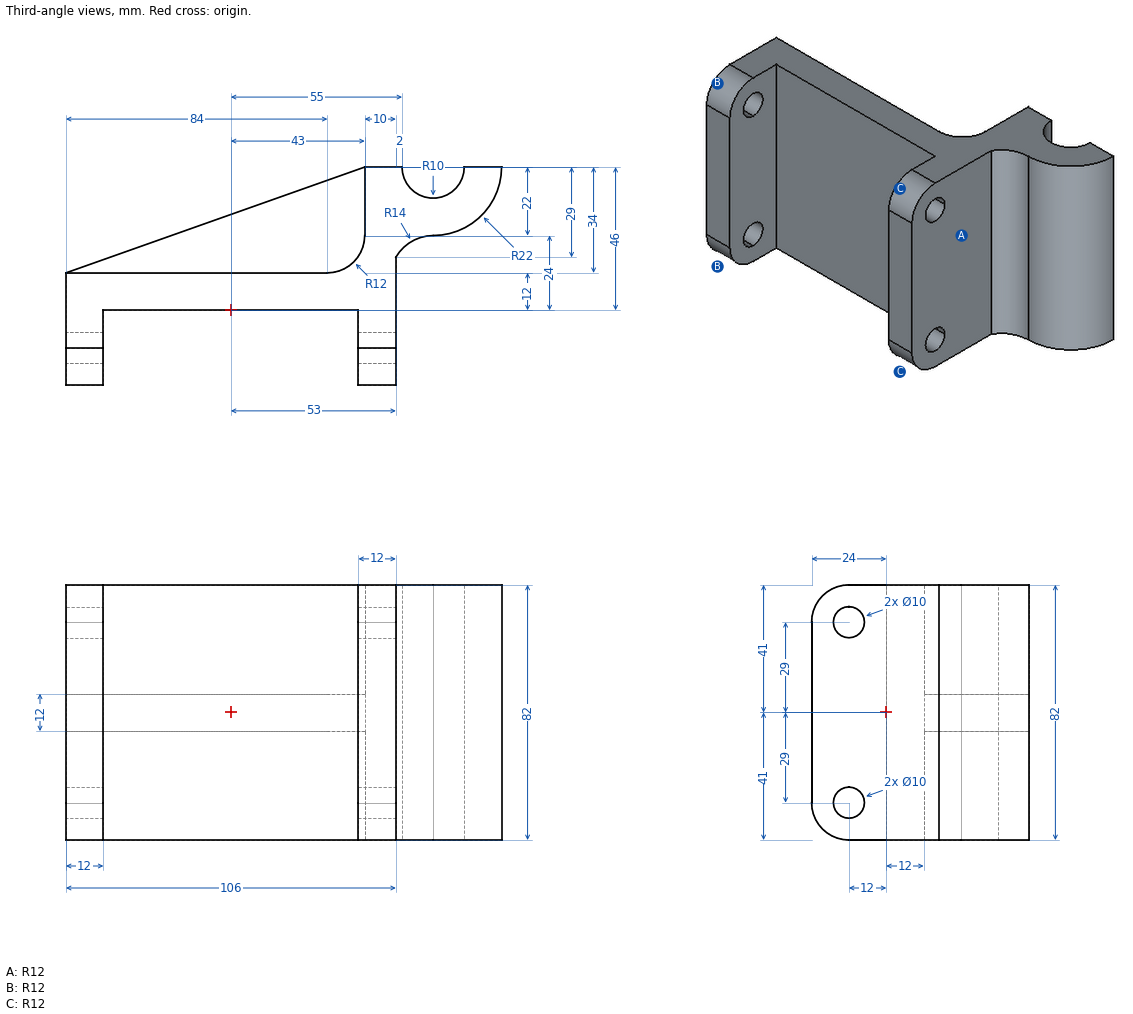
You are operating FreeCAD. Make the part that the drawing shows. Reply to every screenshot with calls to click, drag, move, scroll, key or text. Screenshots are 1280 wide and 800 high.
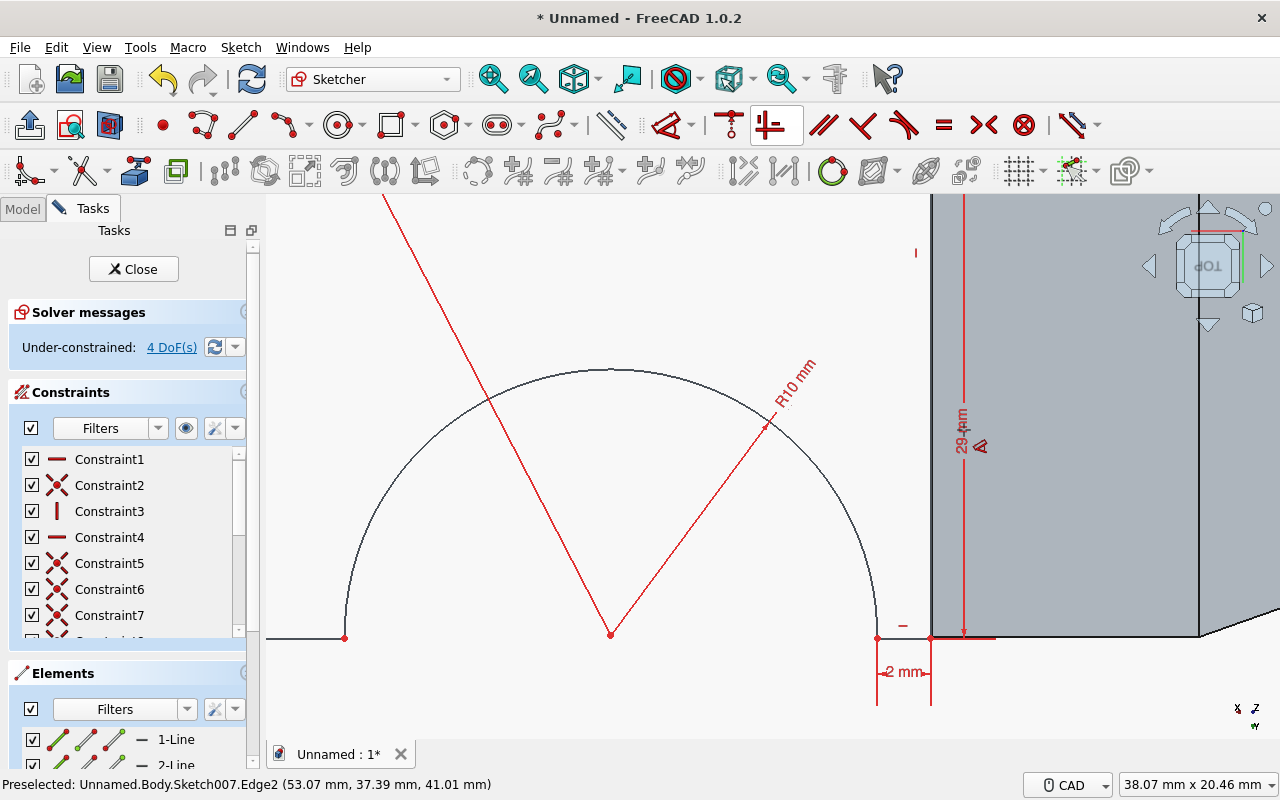
click(877, 639)
click(996, 673)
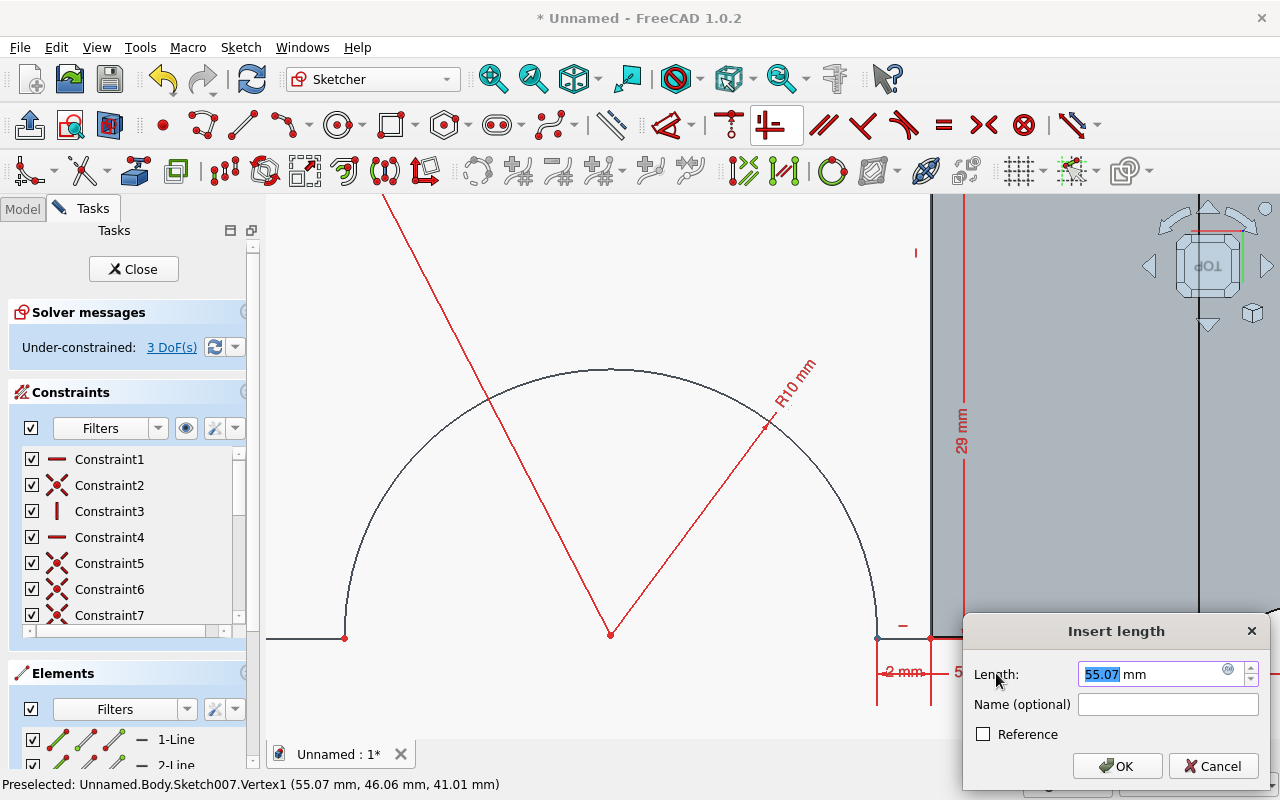
text(55)
key(Return)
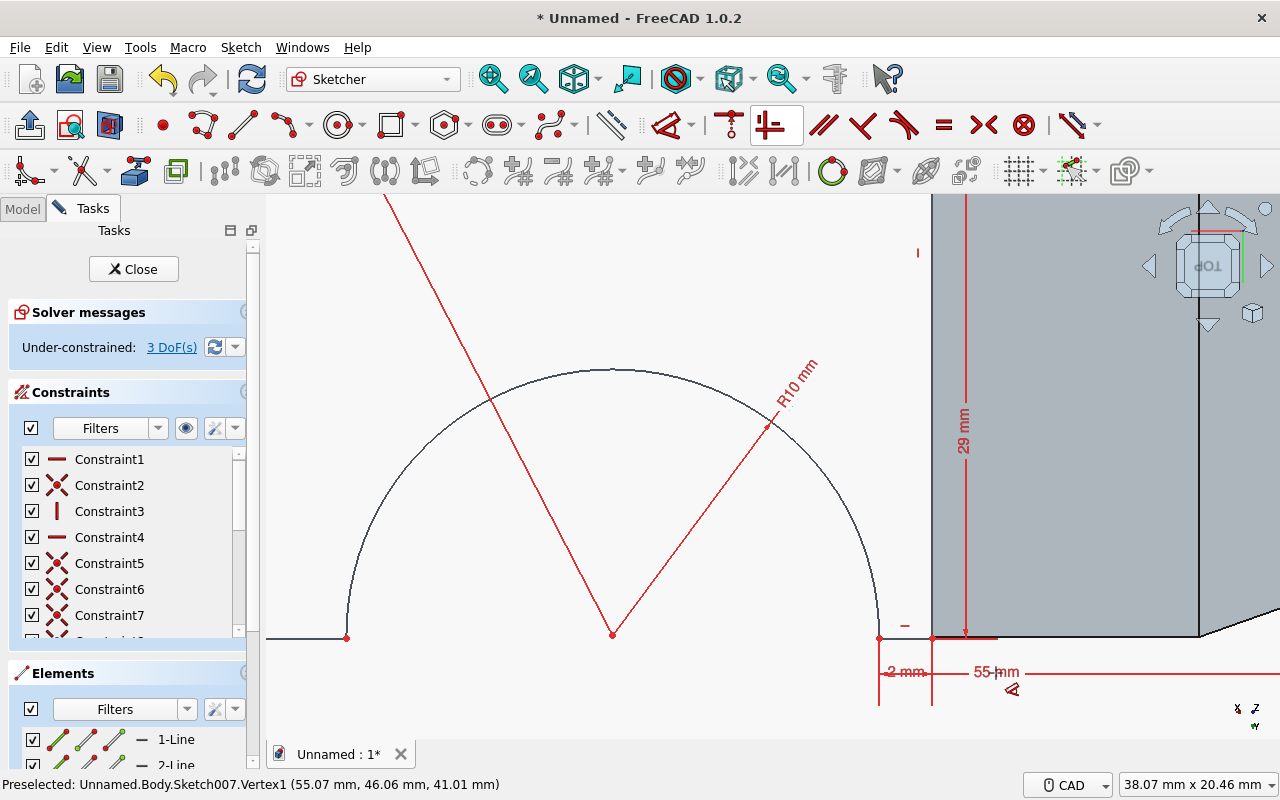
click(879, 639)
click(845, 430)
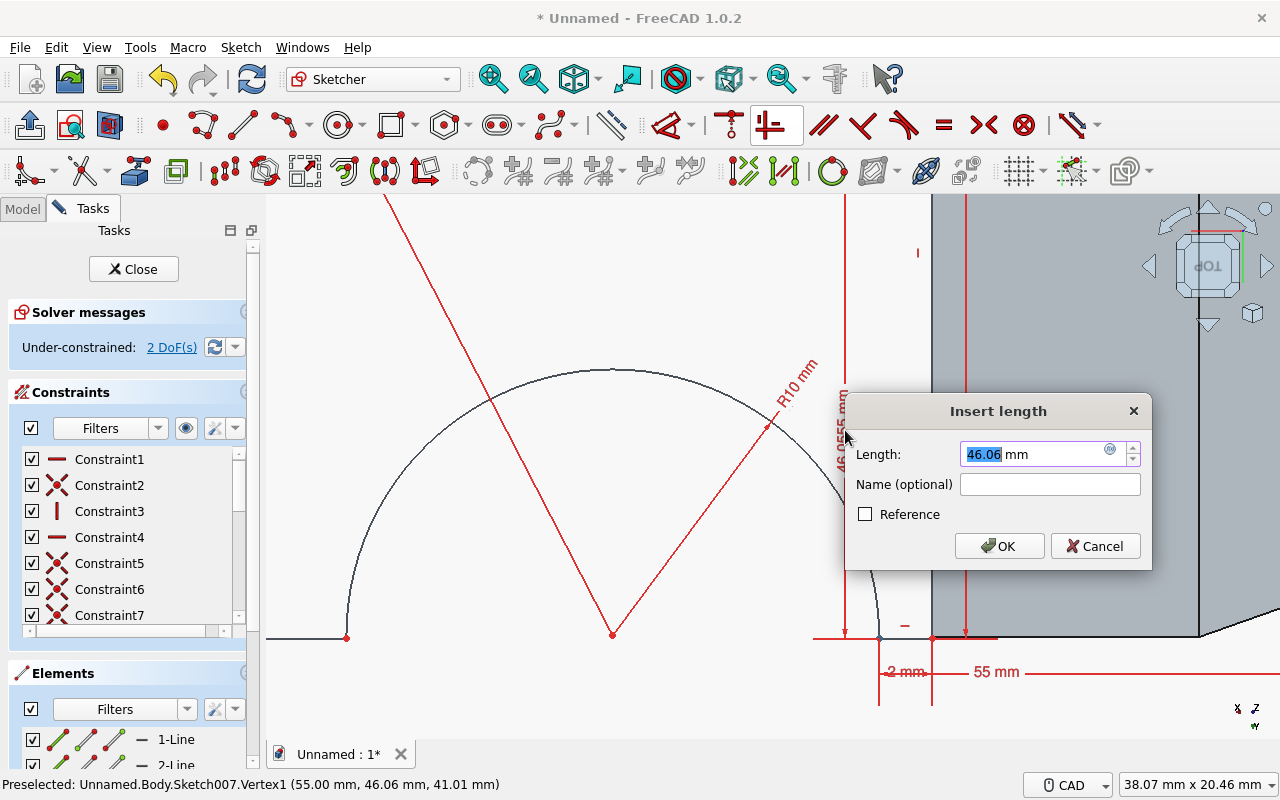
text(46)
key(Return)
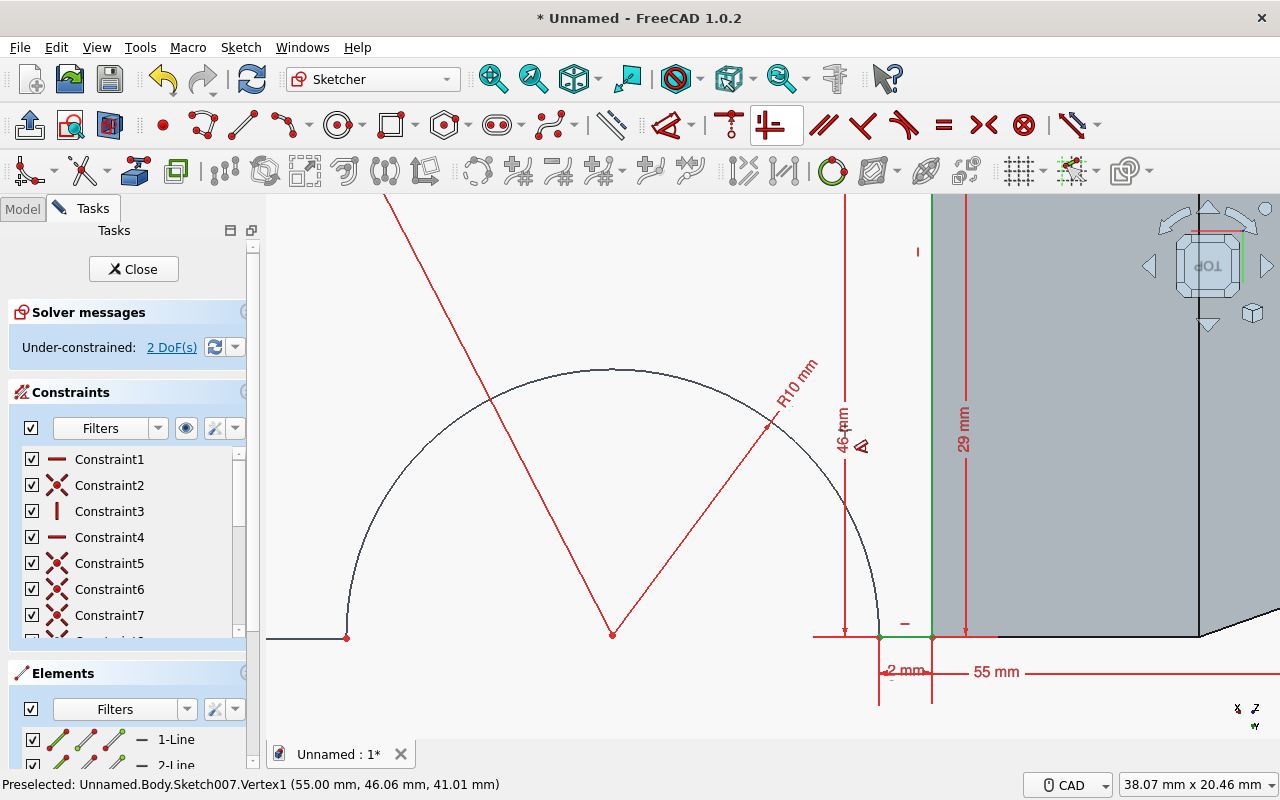
scroll(888, 642, down, 4)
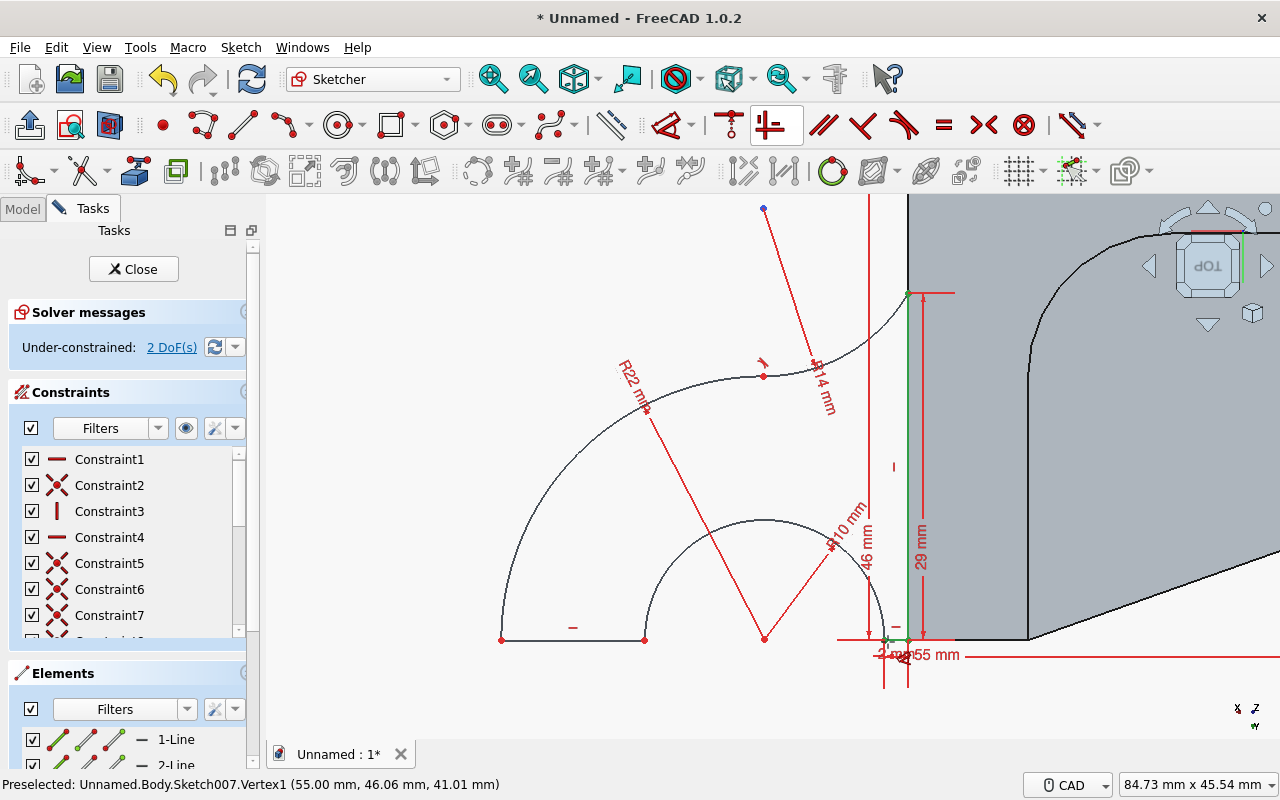
click(501, 641)
click(467, 431)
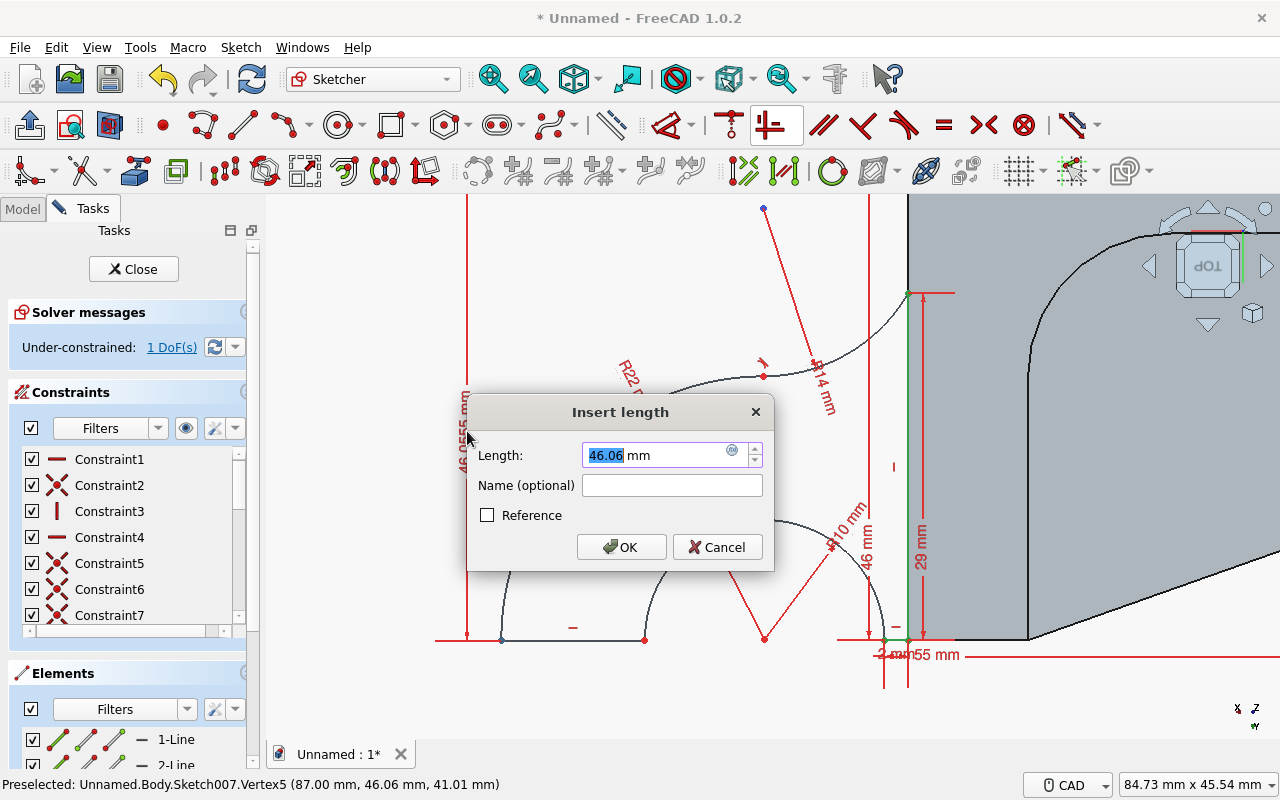
text(46)
key(Return)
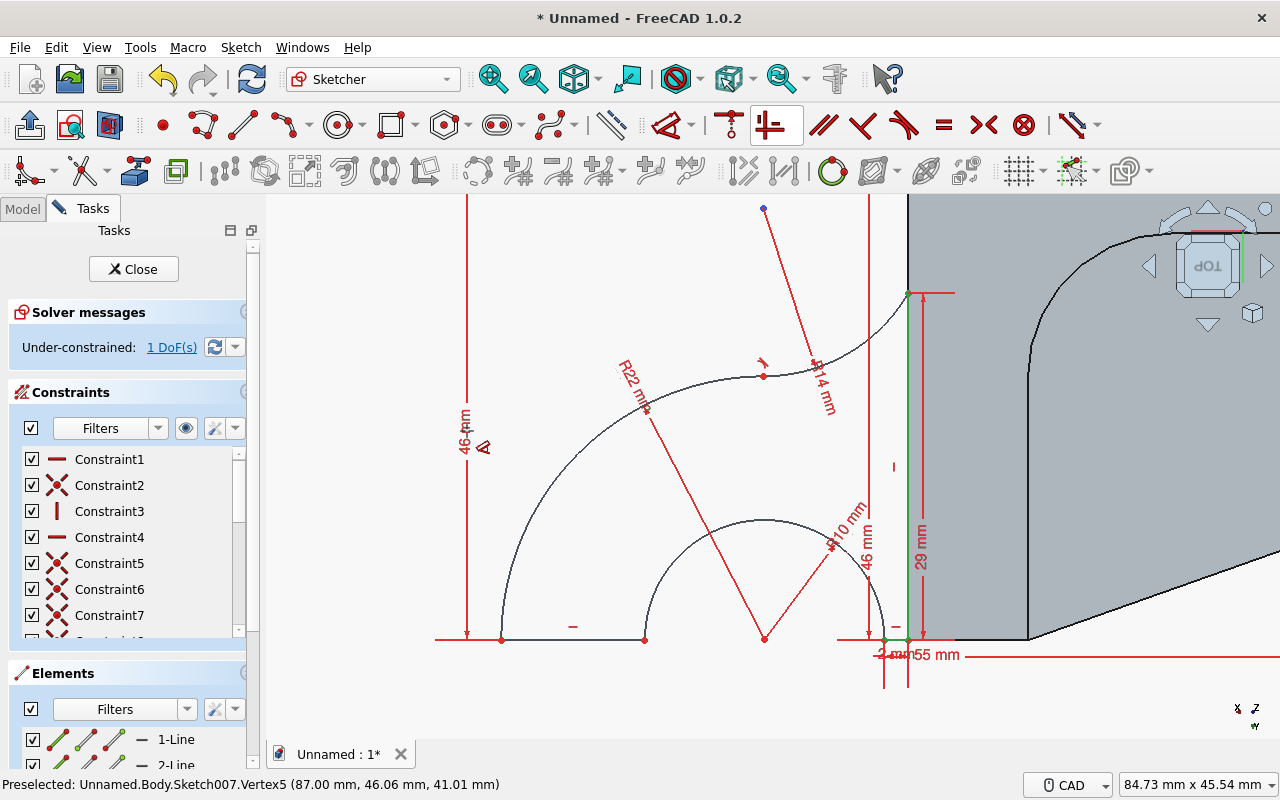
click(765, 640)
click(731, 431)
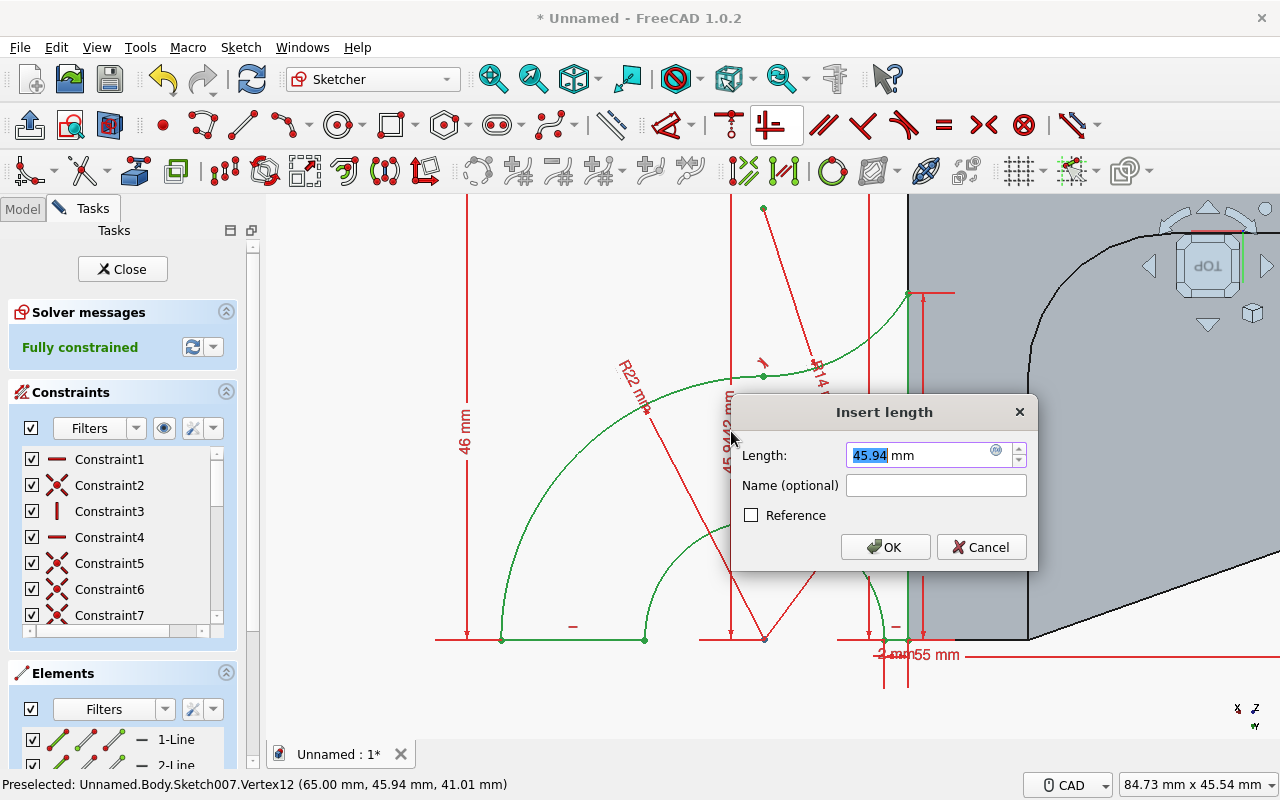
text(46)
key(Return)
key(Escape)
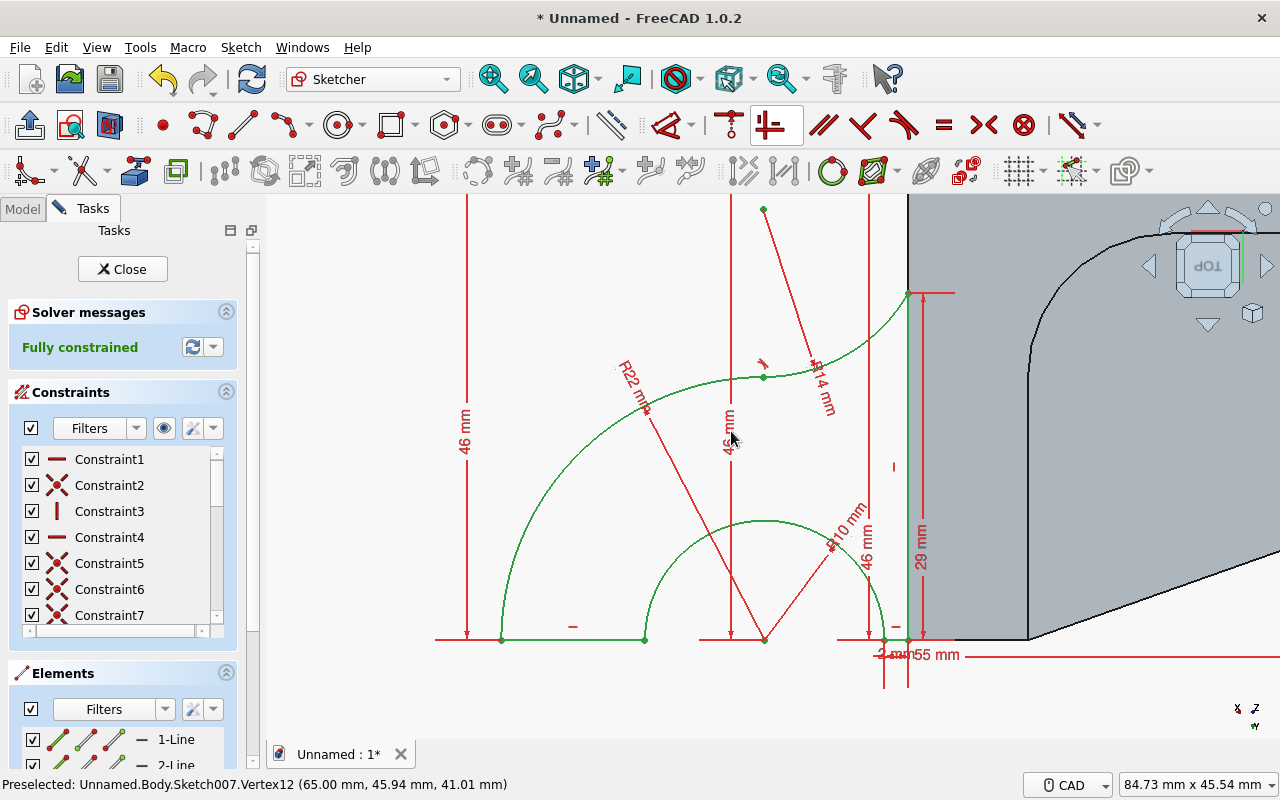
click(123, 269)